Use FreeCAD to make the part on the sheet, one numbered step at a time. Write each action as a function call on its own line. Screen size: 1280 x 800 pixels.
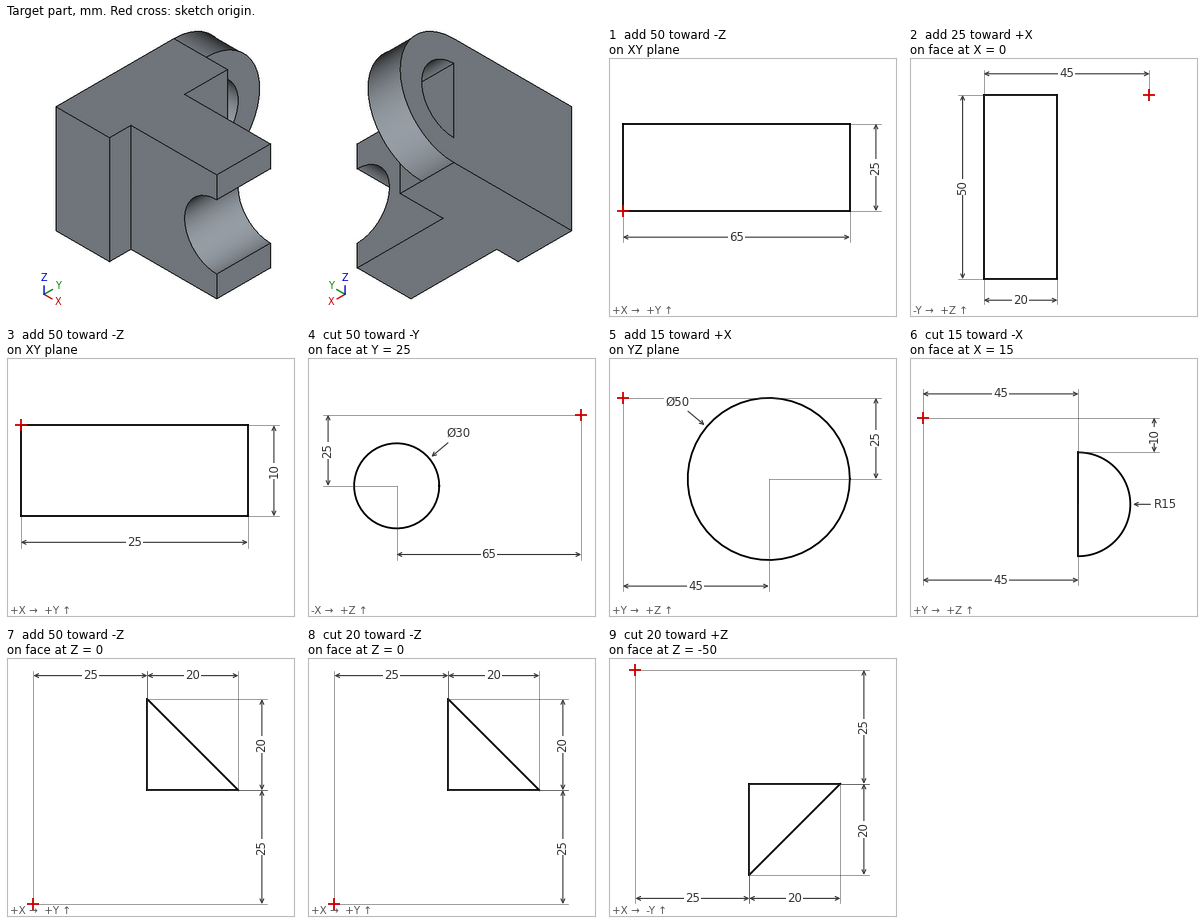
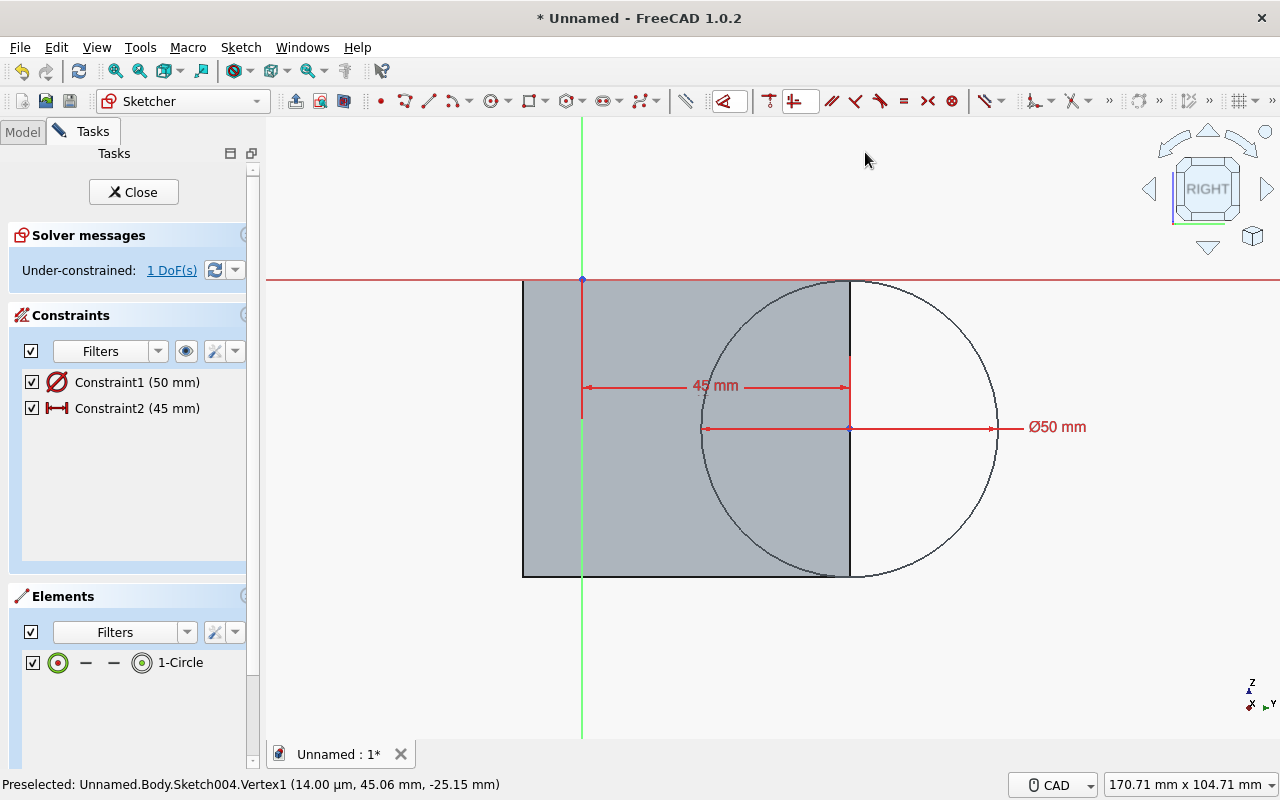
click(850, 429)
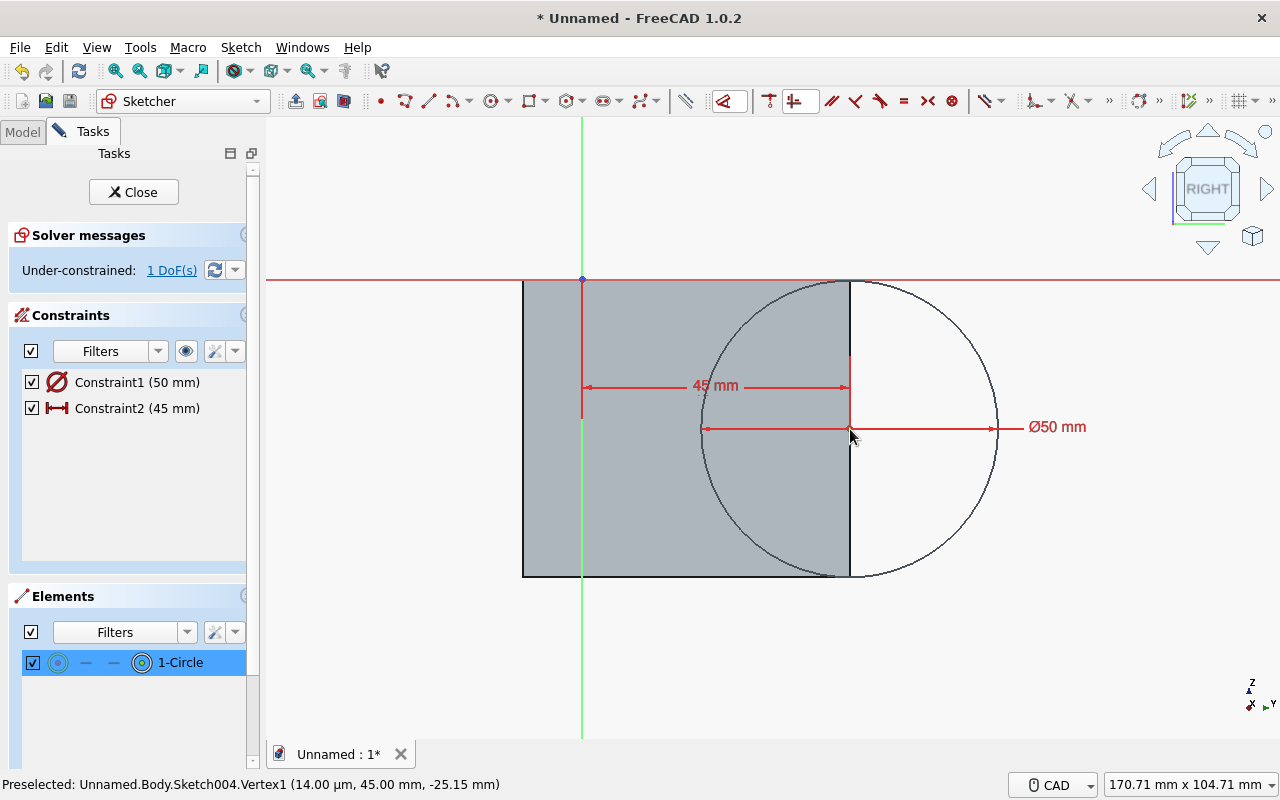
click(742, 102)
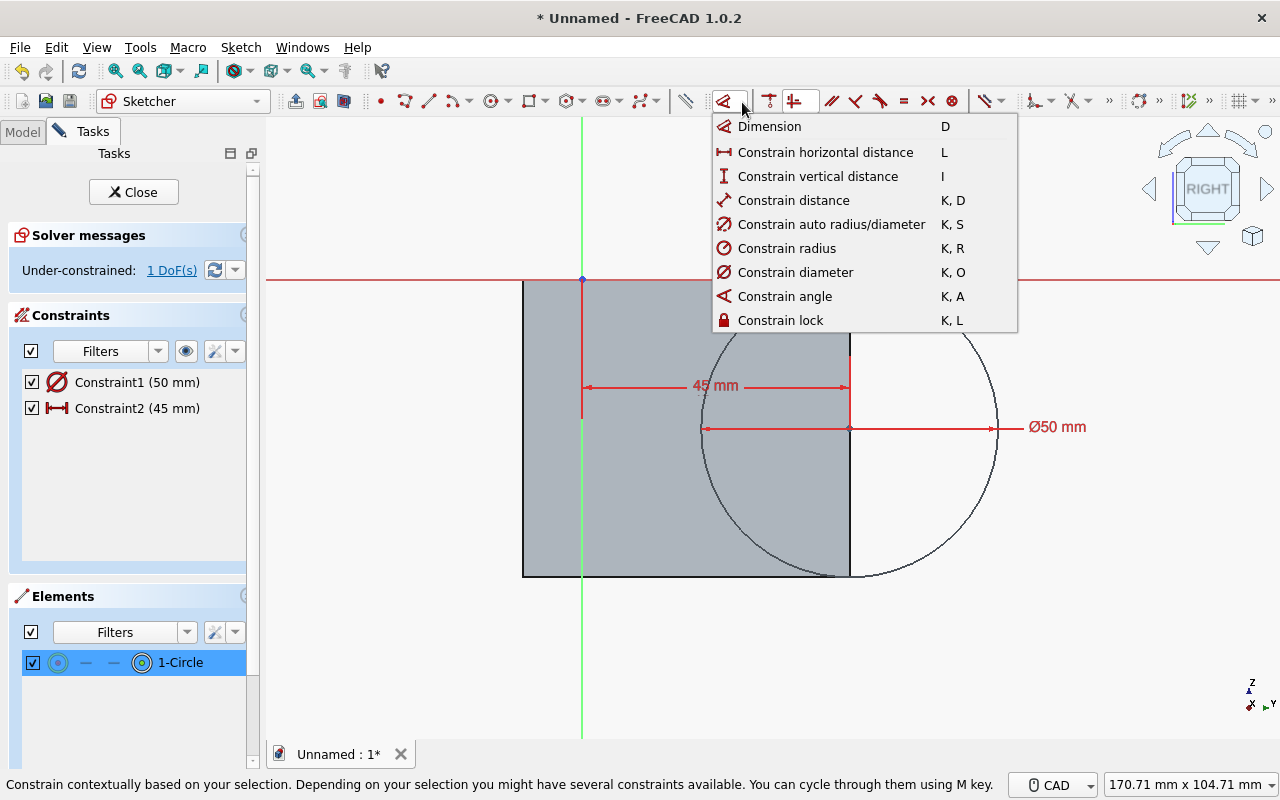
click(865, 176)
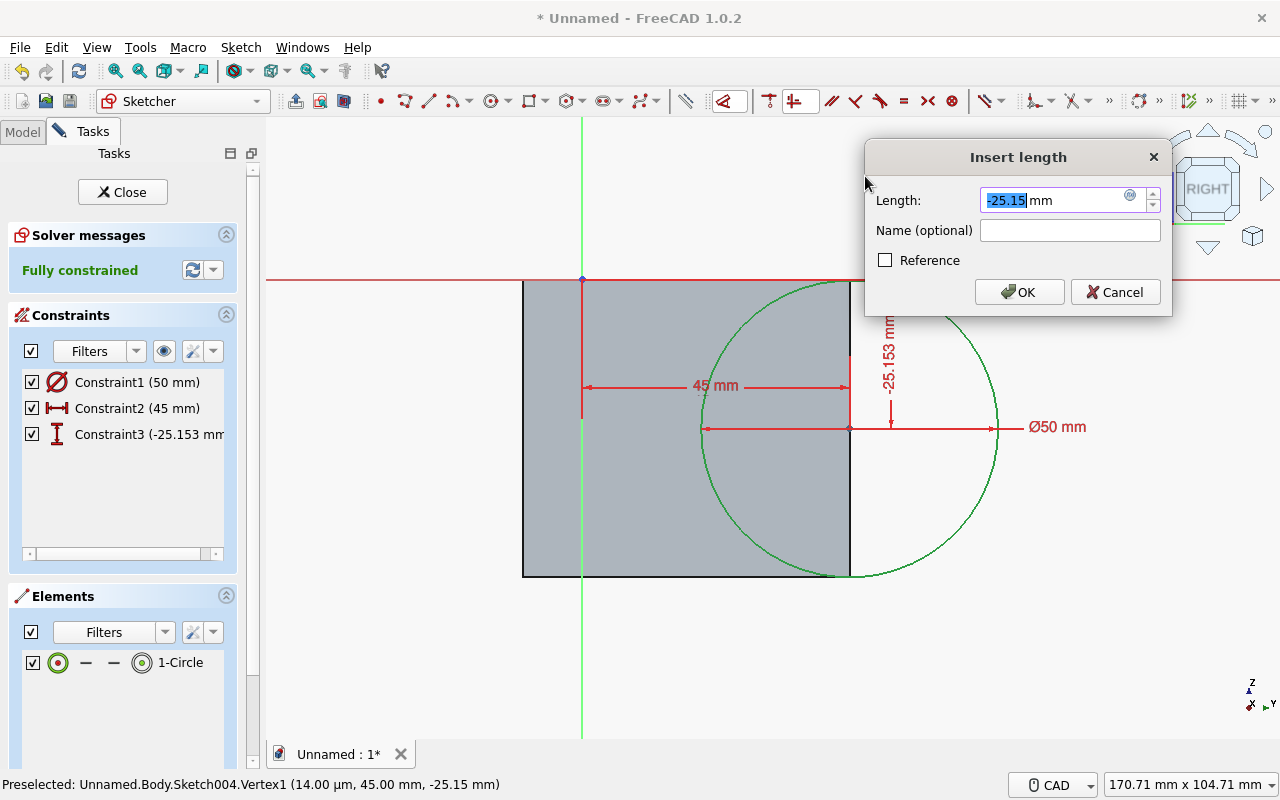
text(-25)
key(Return)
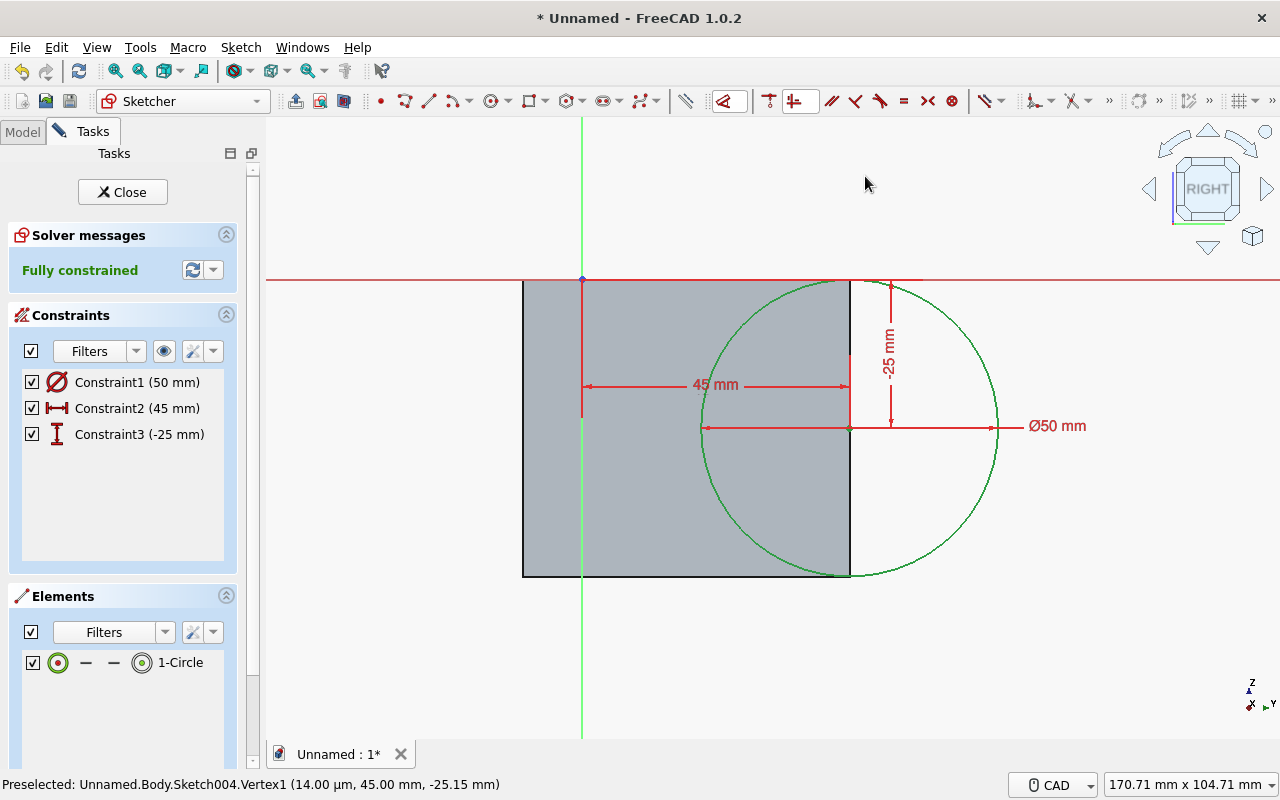
click(123, 192)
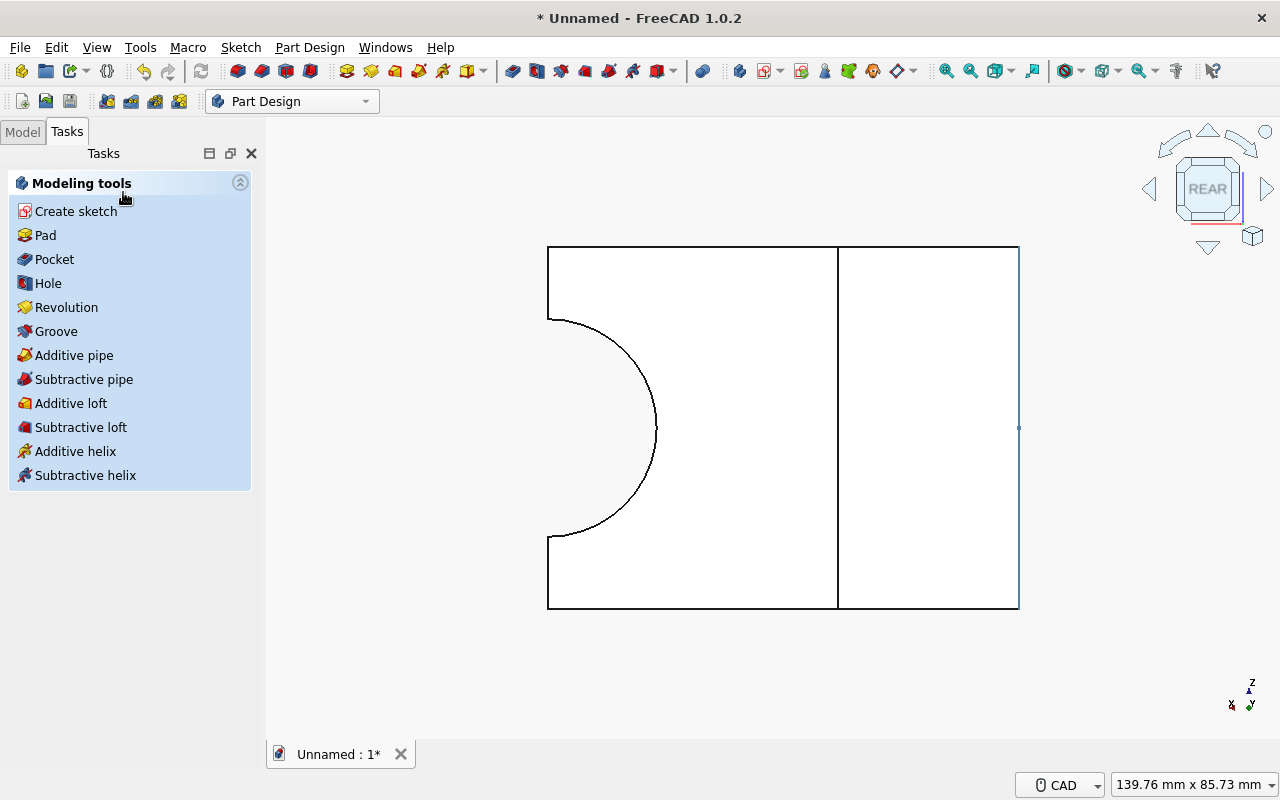
click(348, 72)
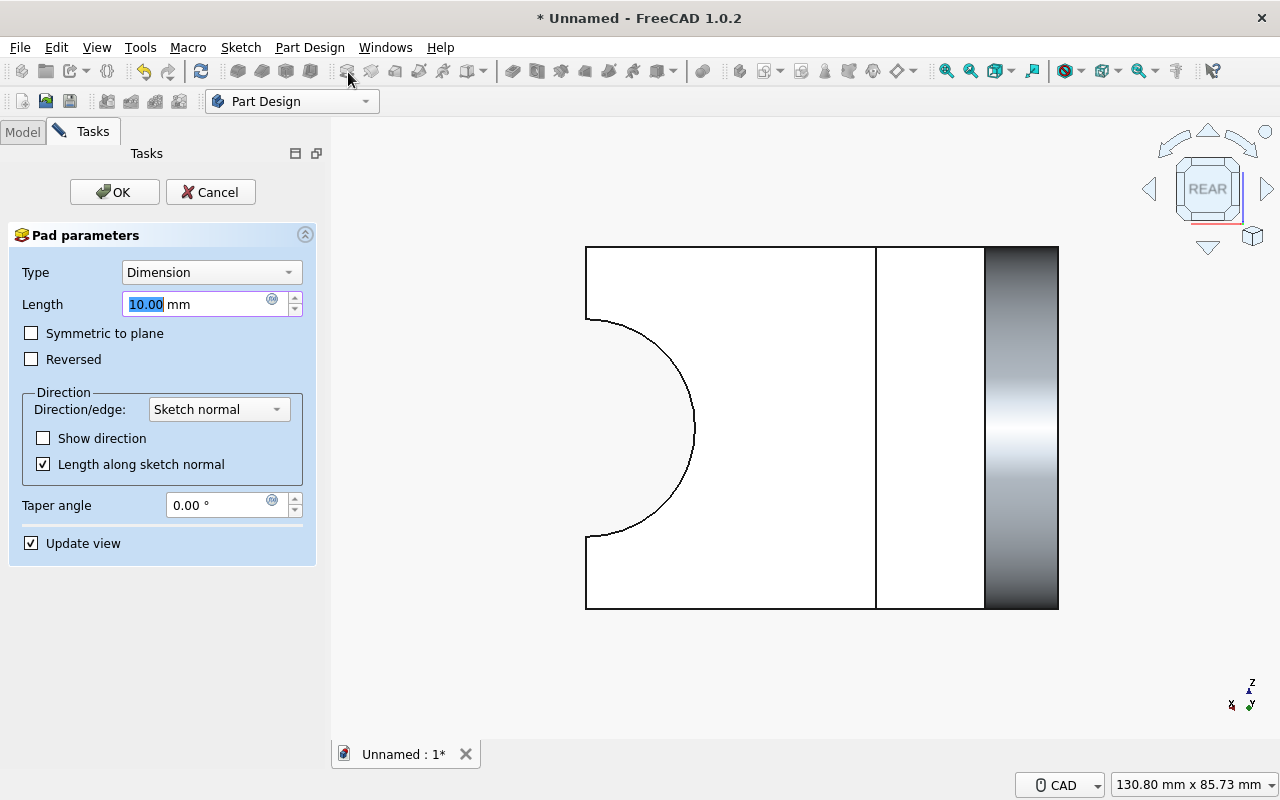
text(15)
key(Tab)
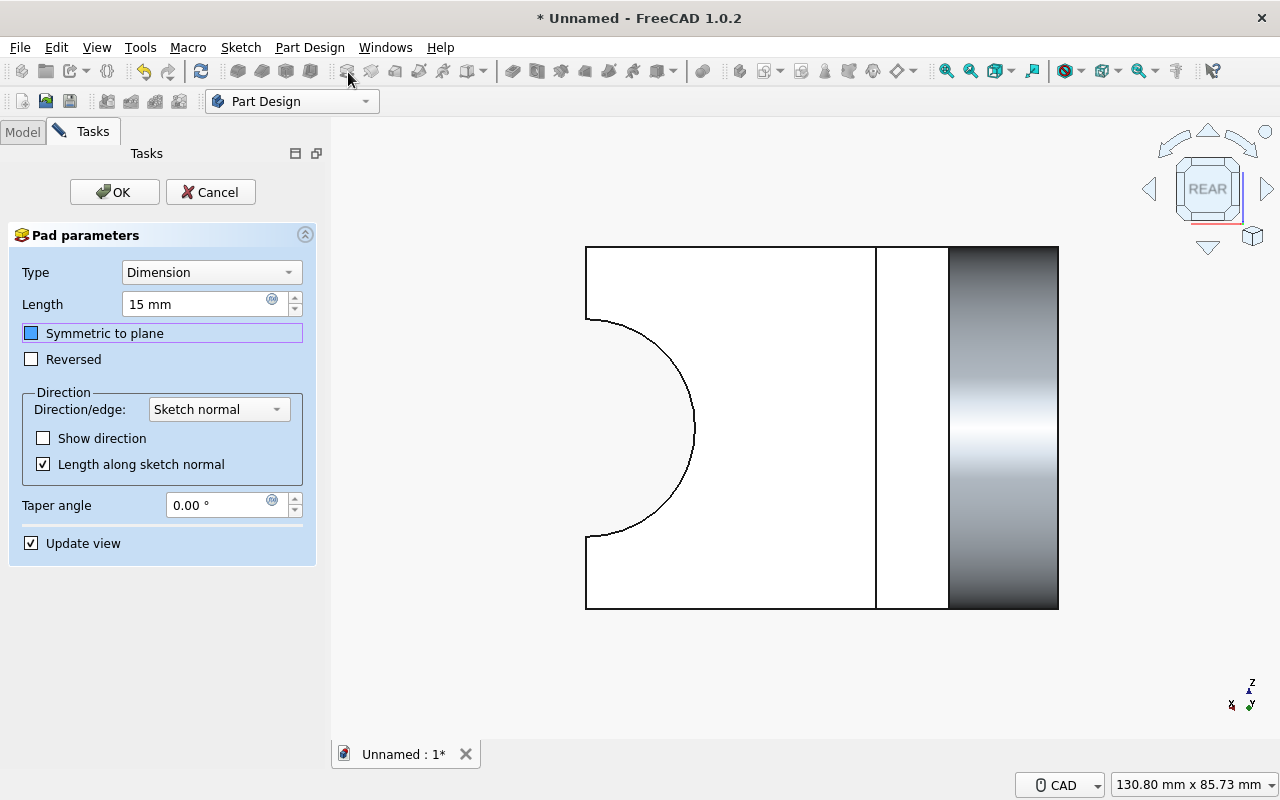
click(115, 192)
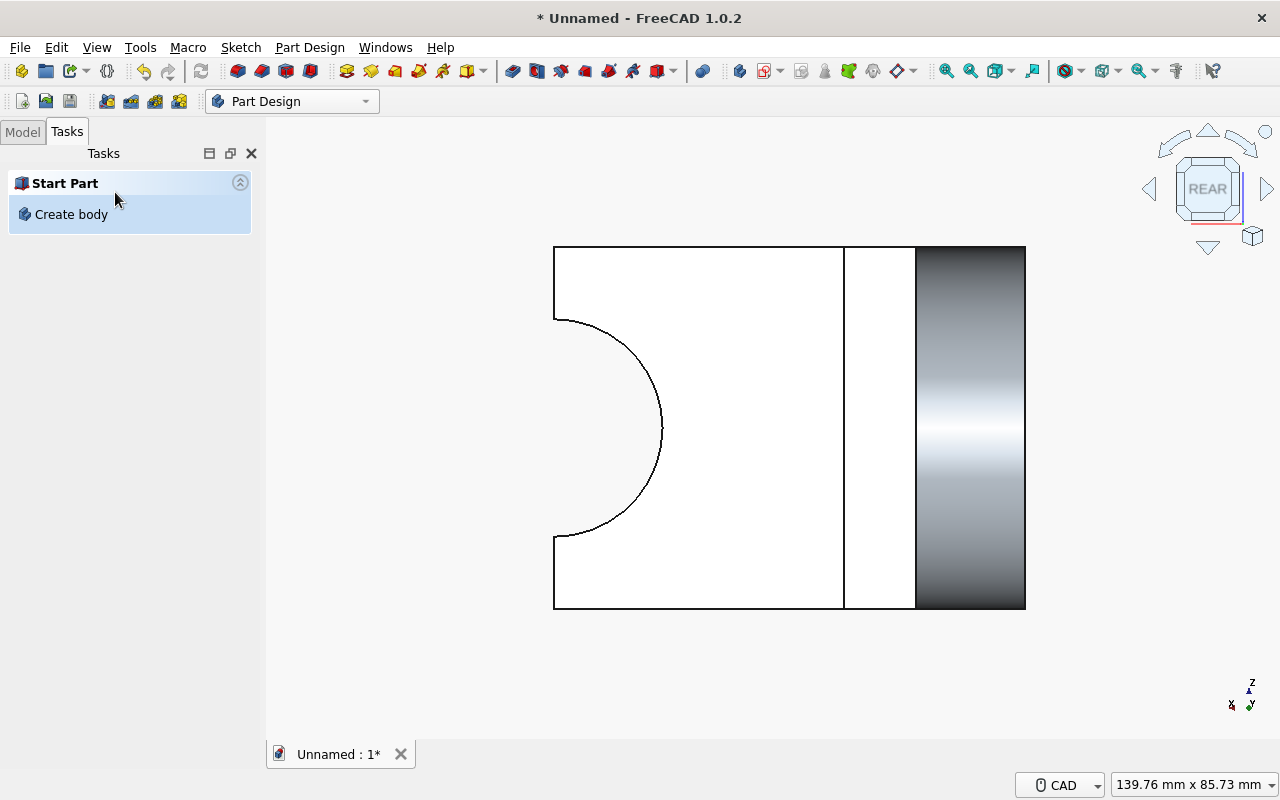
key(0)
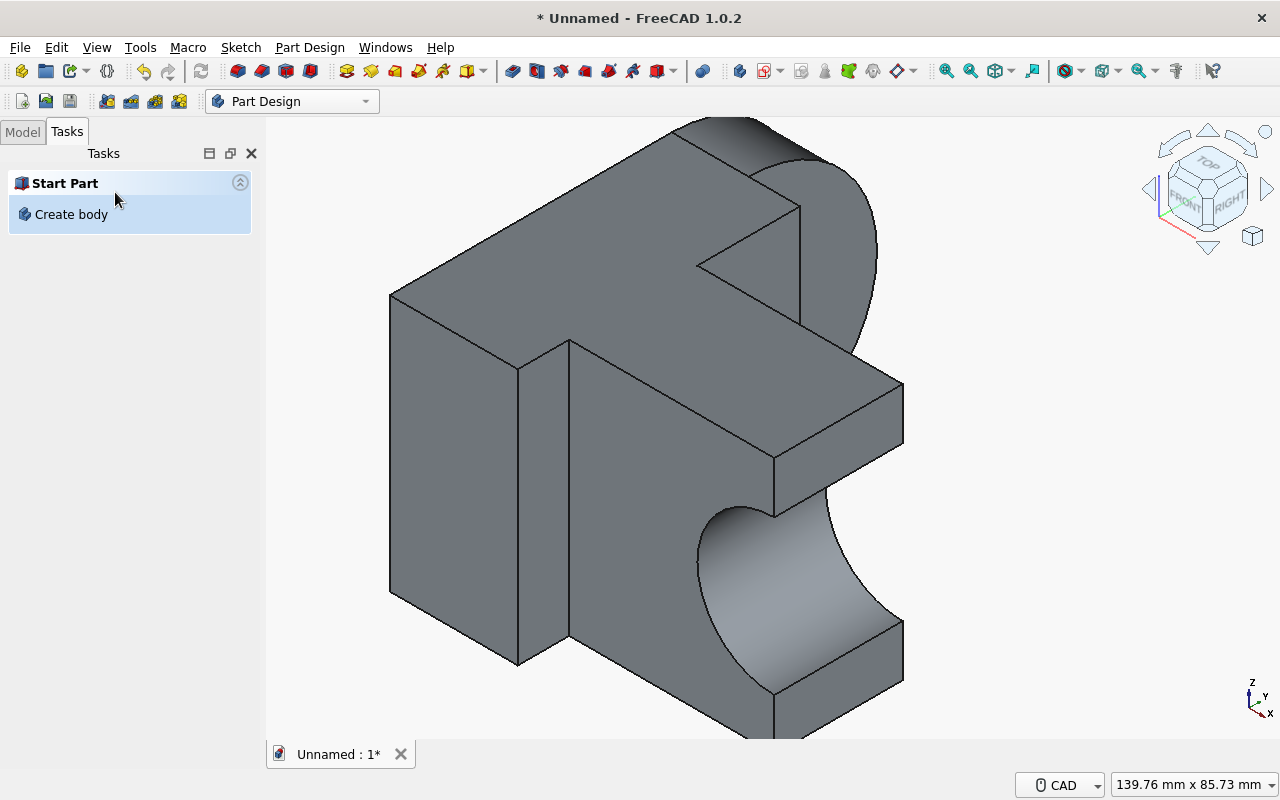
click(948, 72)